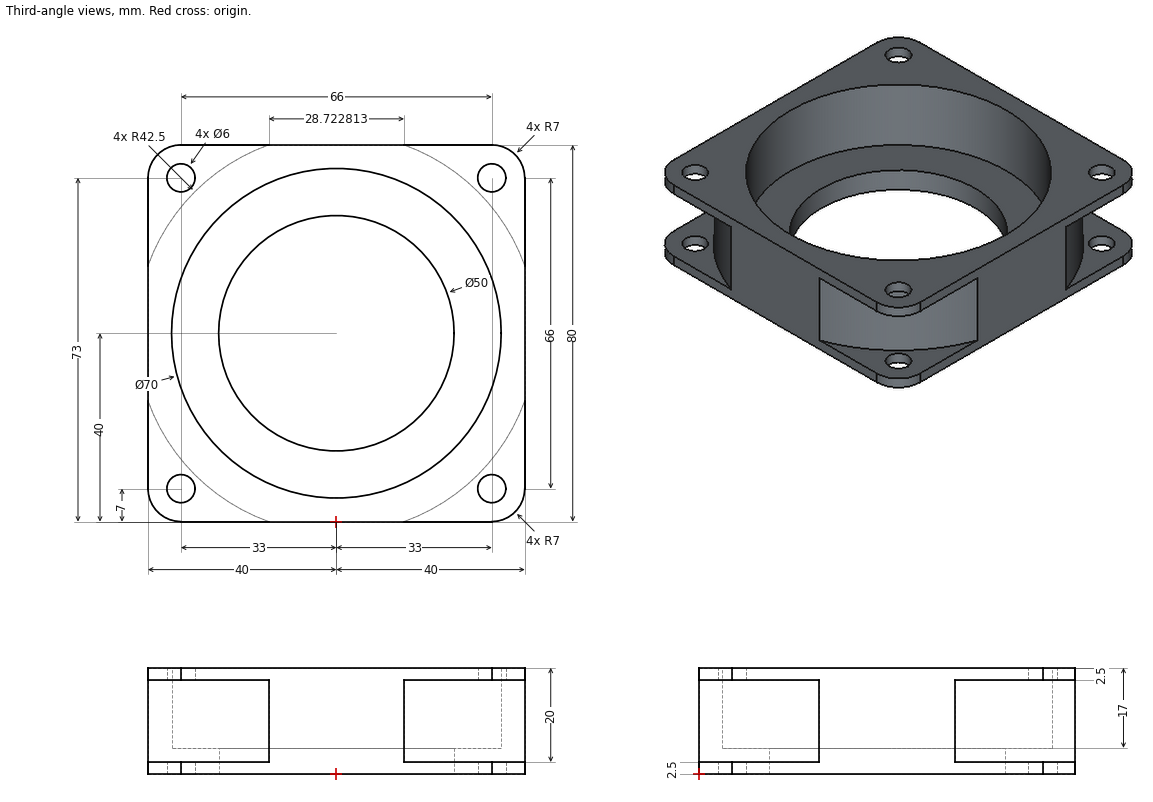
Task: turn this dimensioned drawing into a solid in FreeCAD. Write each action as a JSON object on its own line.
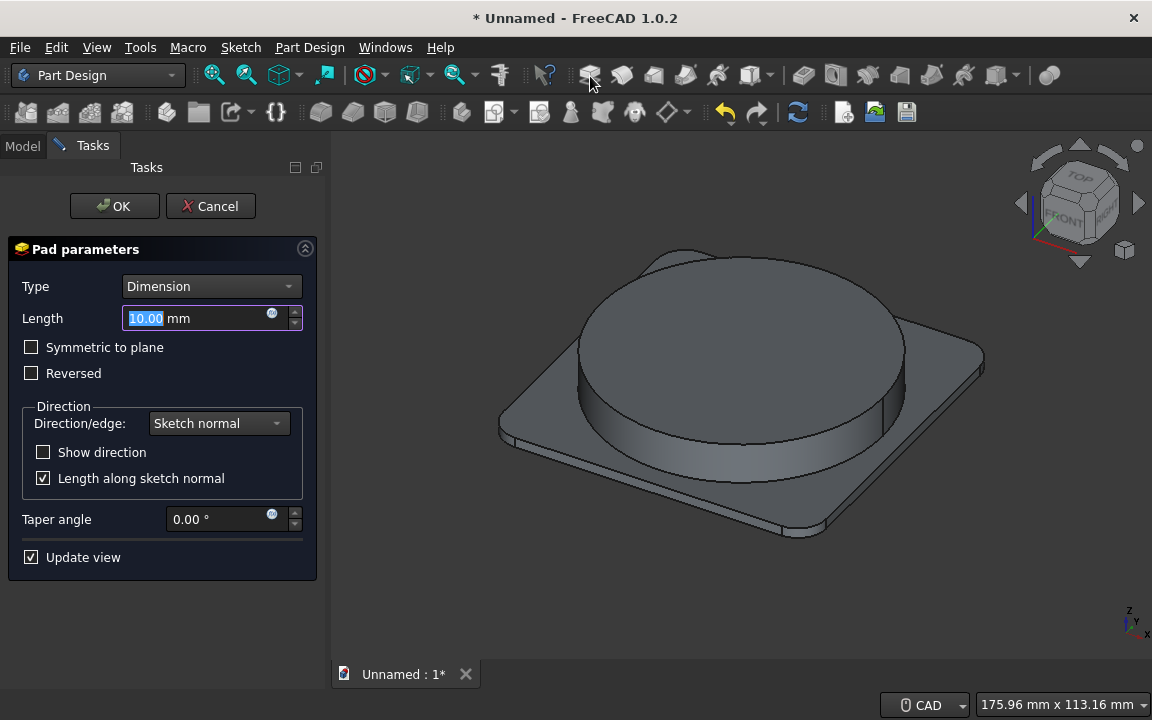
{"action": "type", "text": "20"}
{"action": "key", "text": "Tab"}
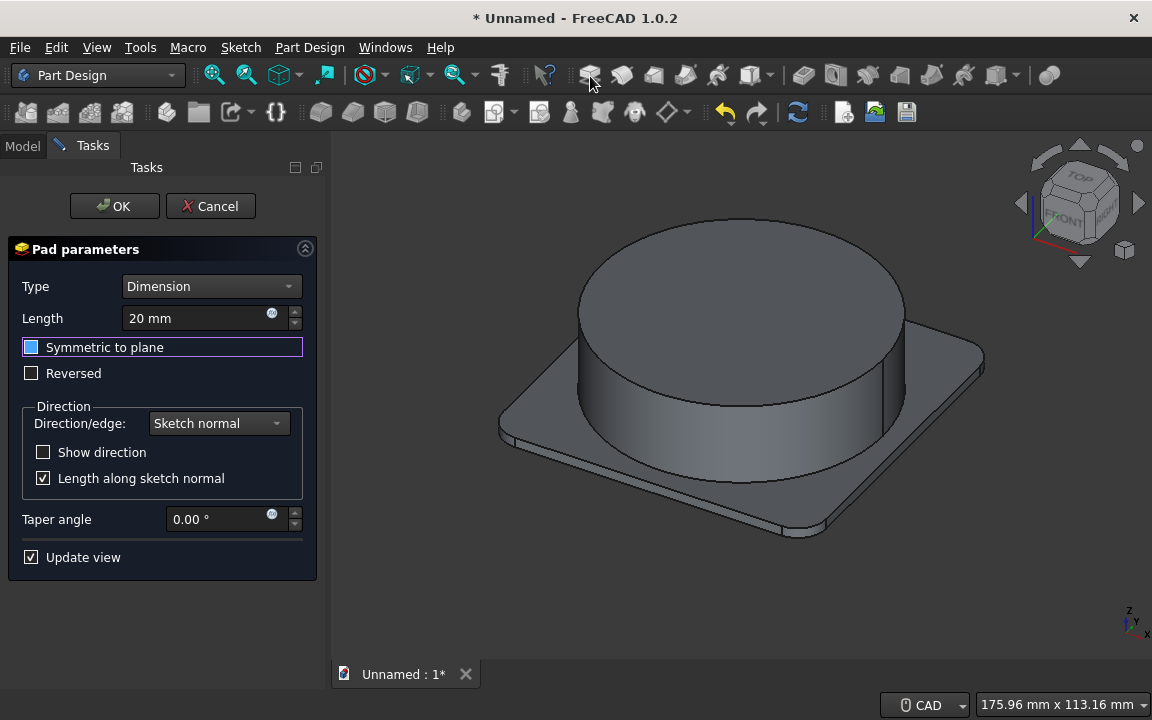
{"action": "left_click", "coordinate": [115, 206]}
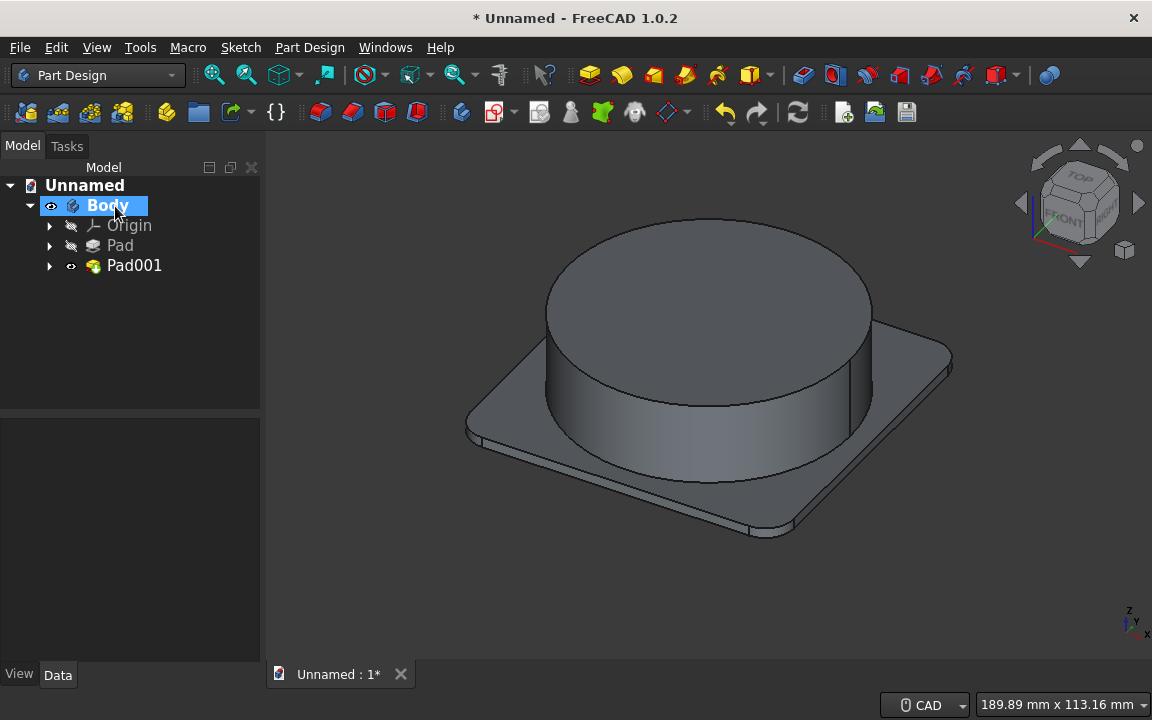
{"action": "left_click", "coordinate": [50, 226]}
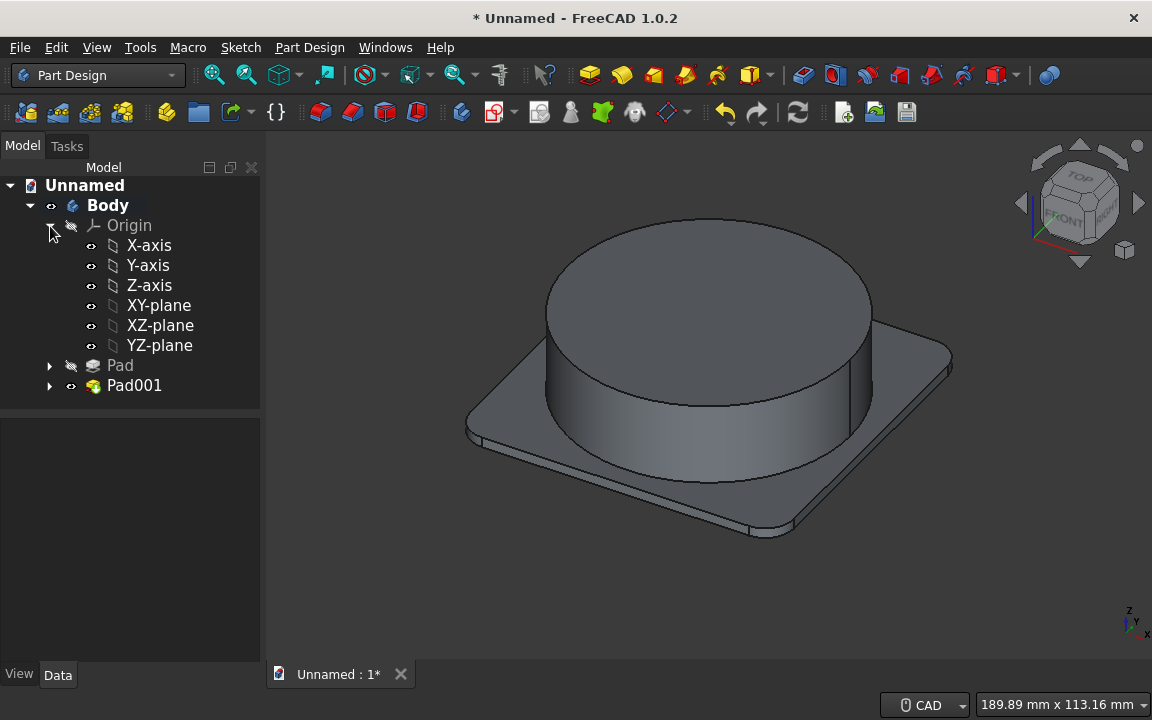
{"action": "left_click", "coordinate": [136, 306]}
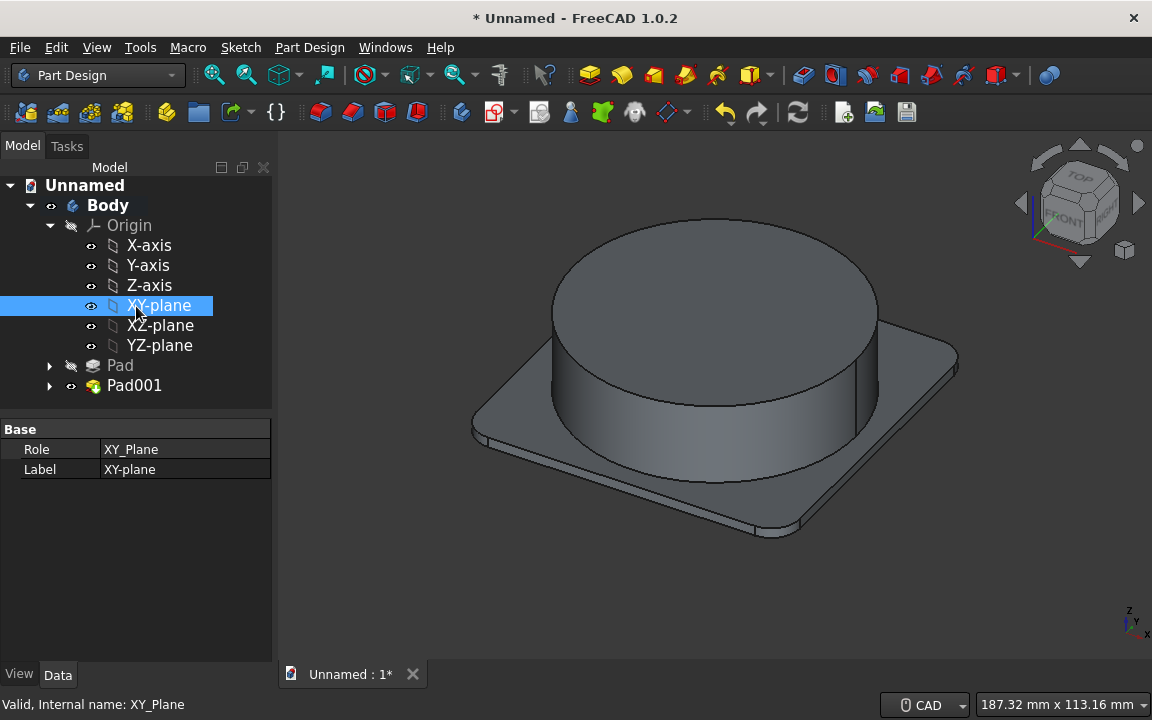
{"action": "left_click", "coordinate": [668, 112]}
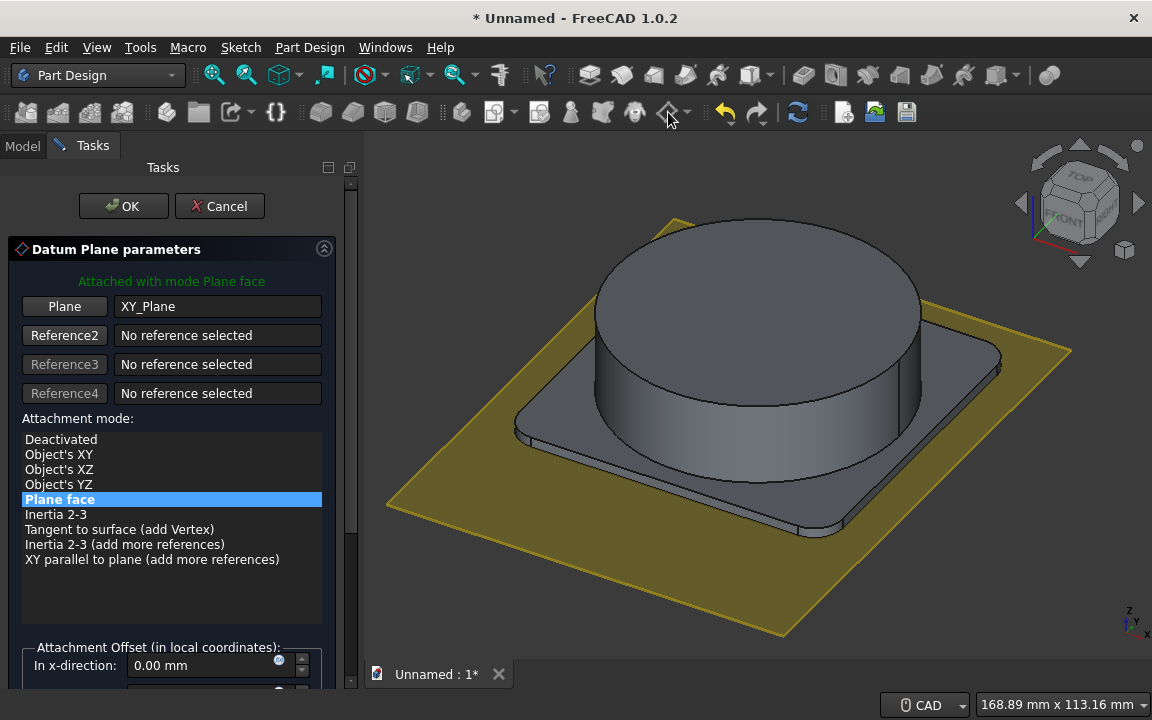
{"action": "scroll", "coordinate": [351, 432], "scroll_direction": "down", "scroll_amount": 2}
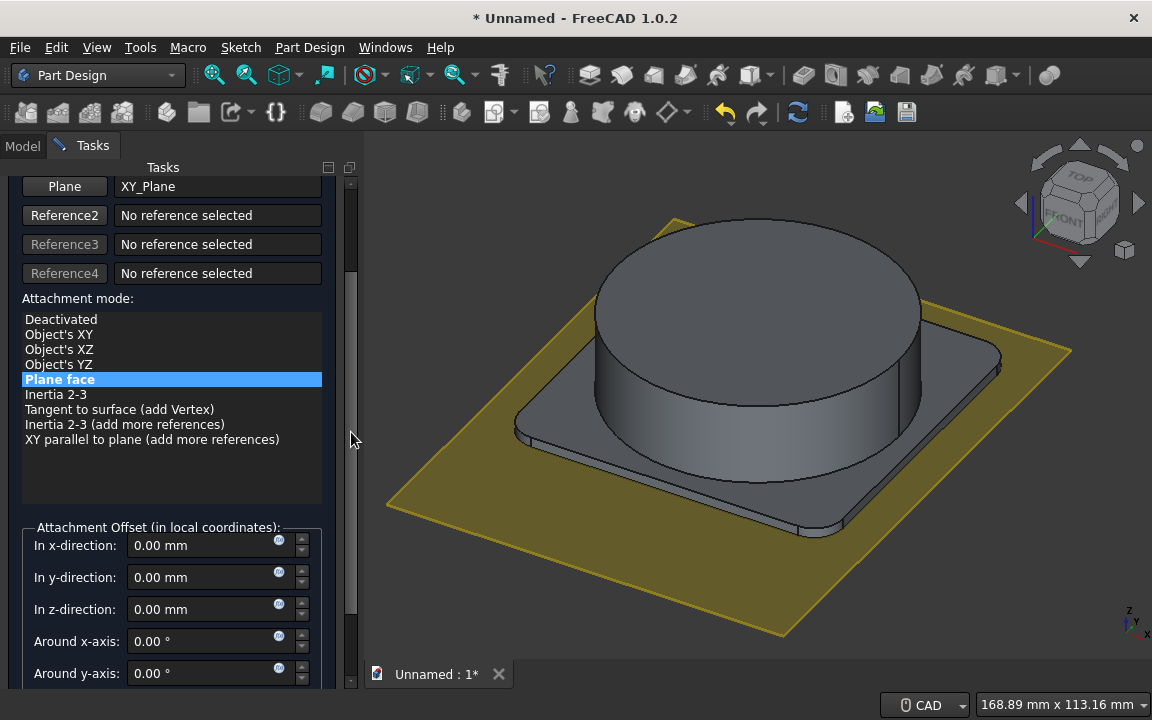
{"action": "triple_click", "coordinate": [210, 609]}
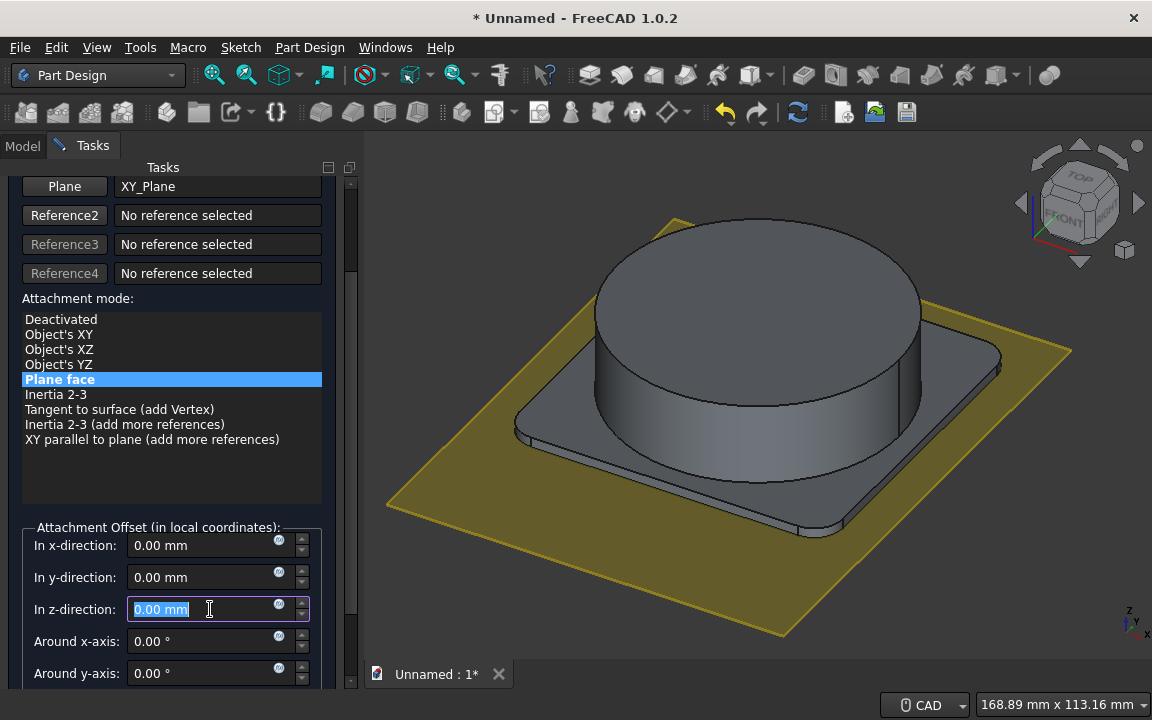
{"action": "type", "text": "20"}
{"action": "key", "text": "Tab"}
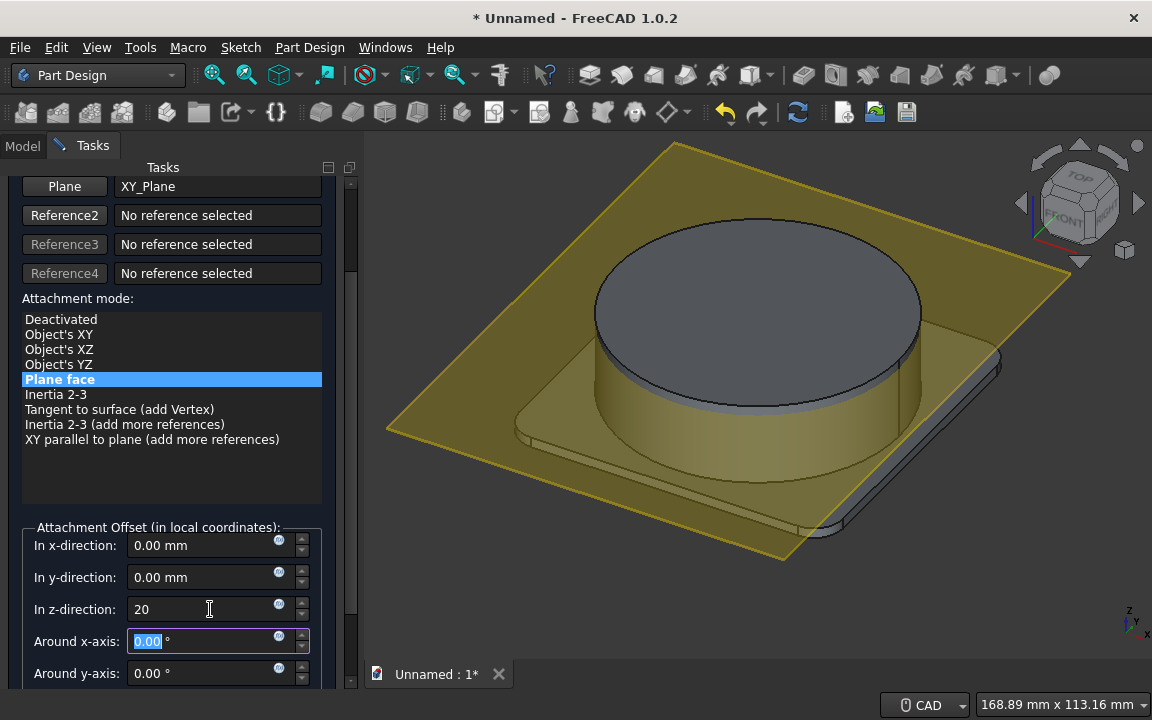
{"action": "scroll", "coordinate": [351, 432], "scroll_direction": "up", "scroll_amount": 3}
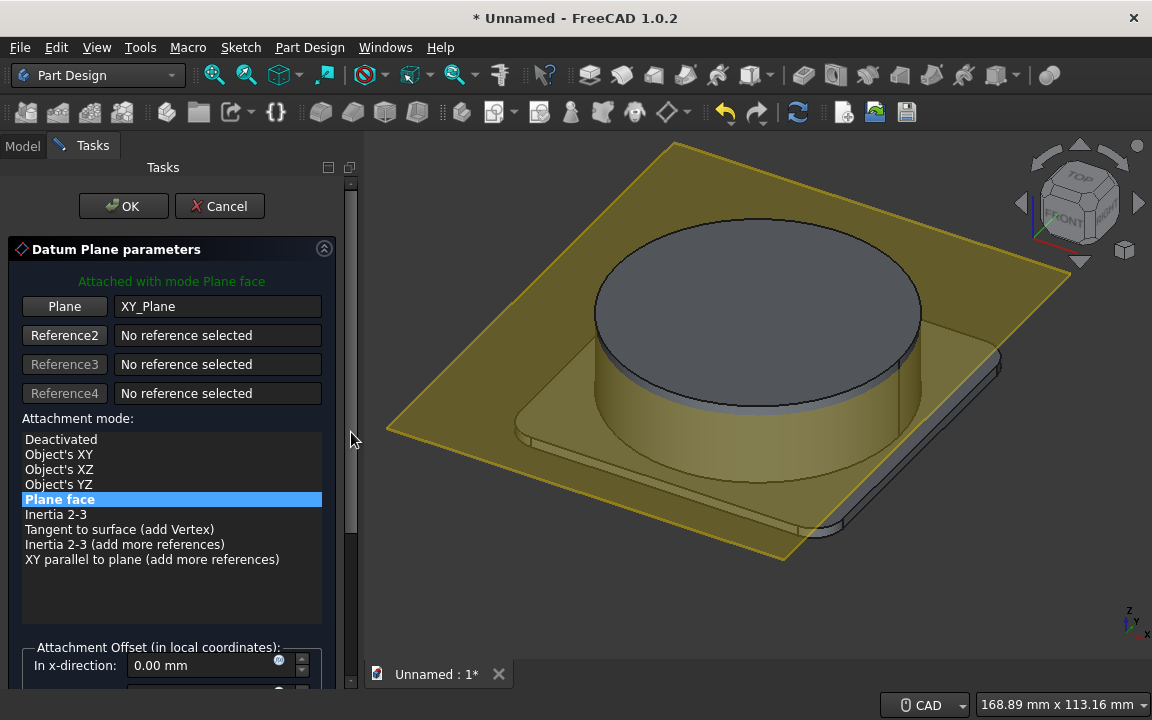
{"action": "left_click", "coordinate": [124, 206]}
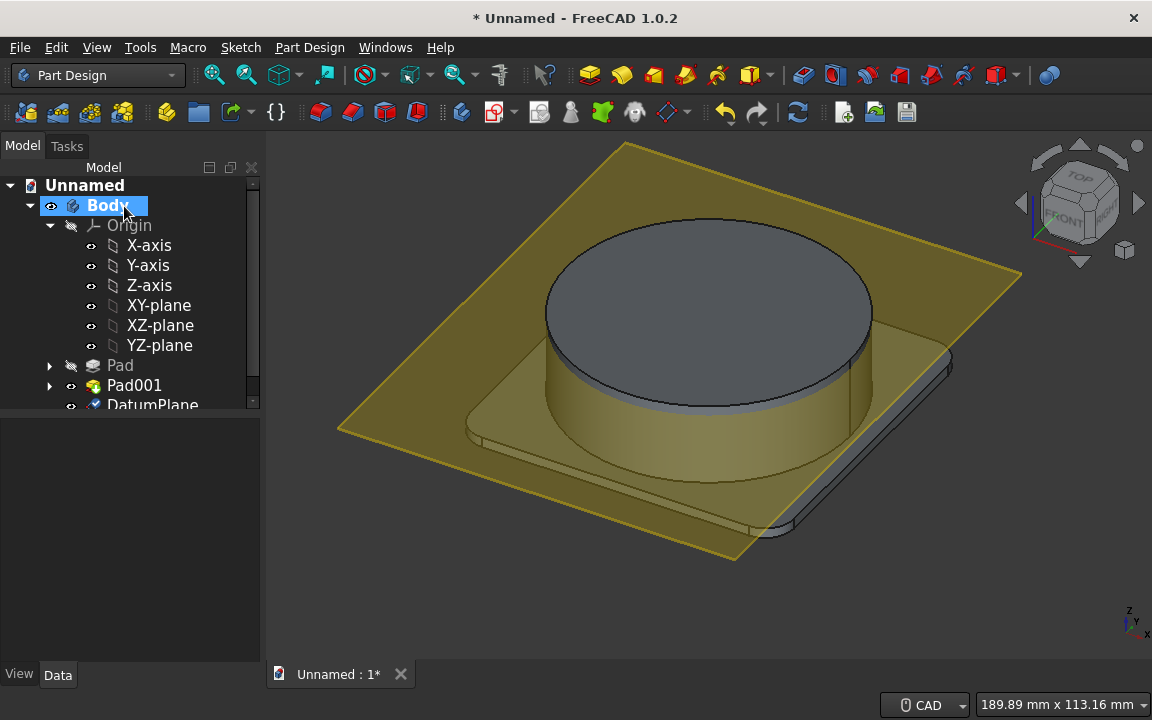
{"action": "left_click", "coordinate": [116, 406]}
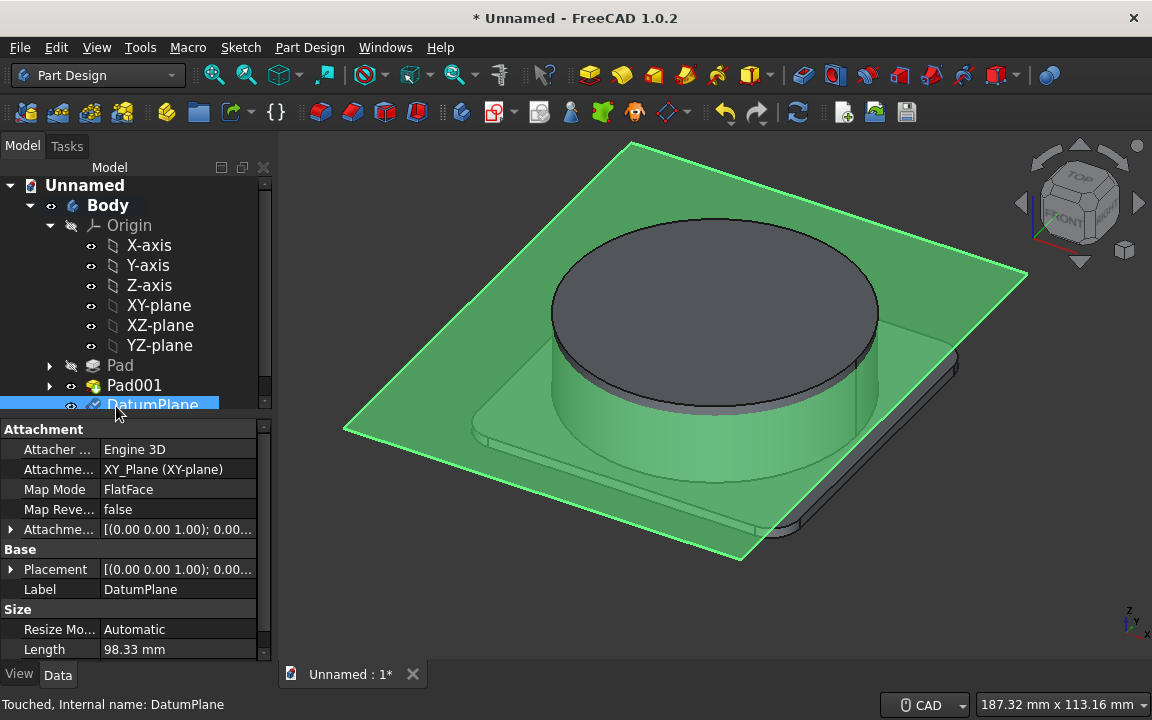
{"action": "left_click", "coordinate": [494, 112]}